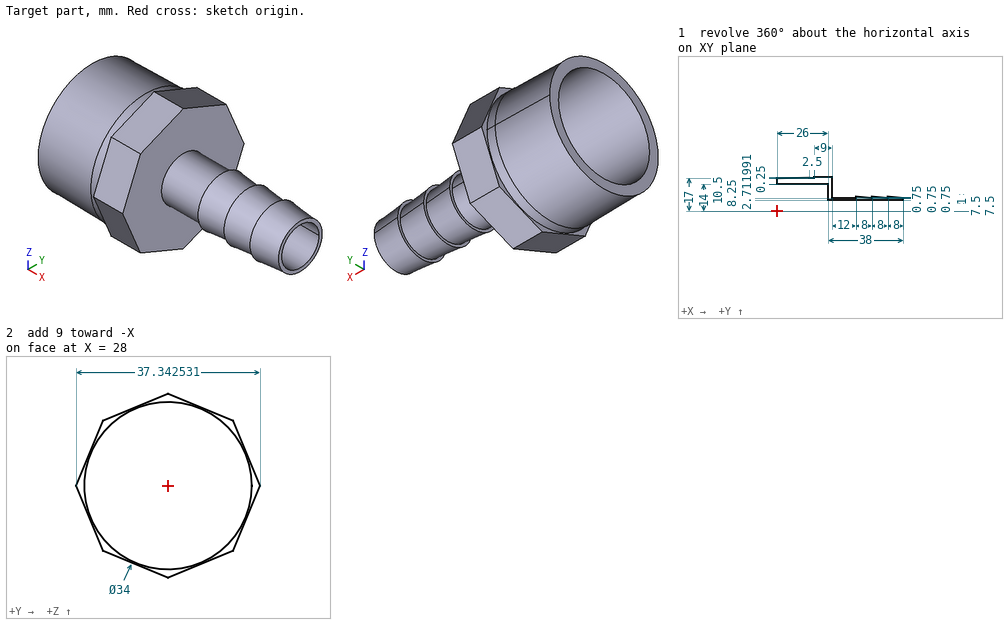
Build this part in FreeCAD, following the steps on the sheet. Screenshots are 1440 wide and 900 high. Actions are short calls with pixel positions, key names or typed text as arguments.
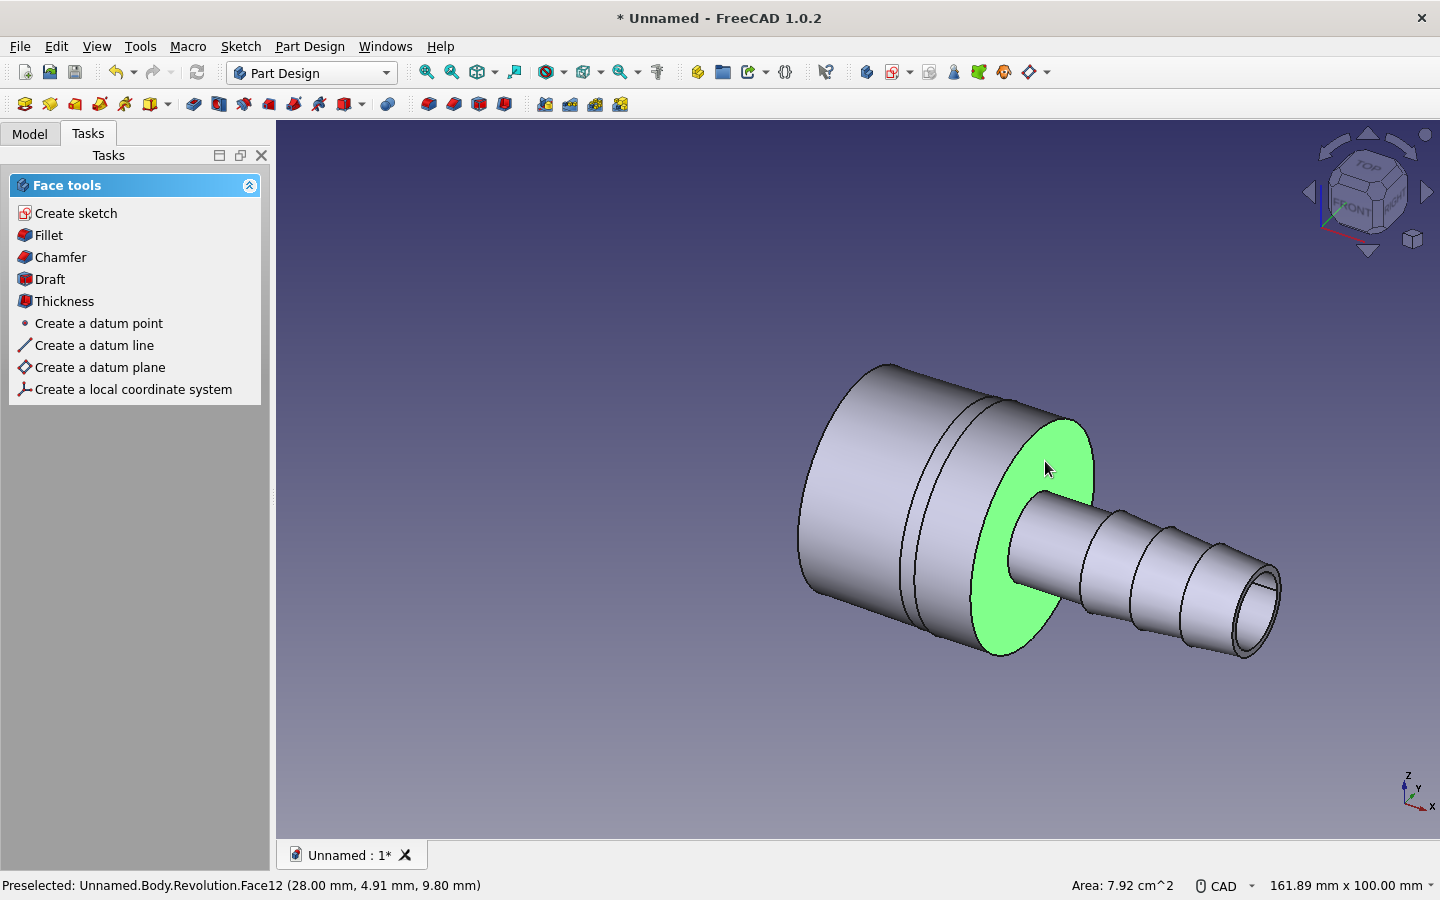
click(892, 72)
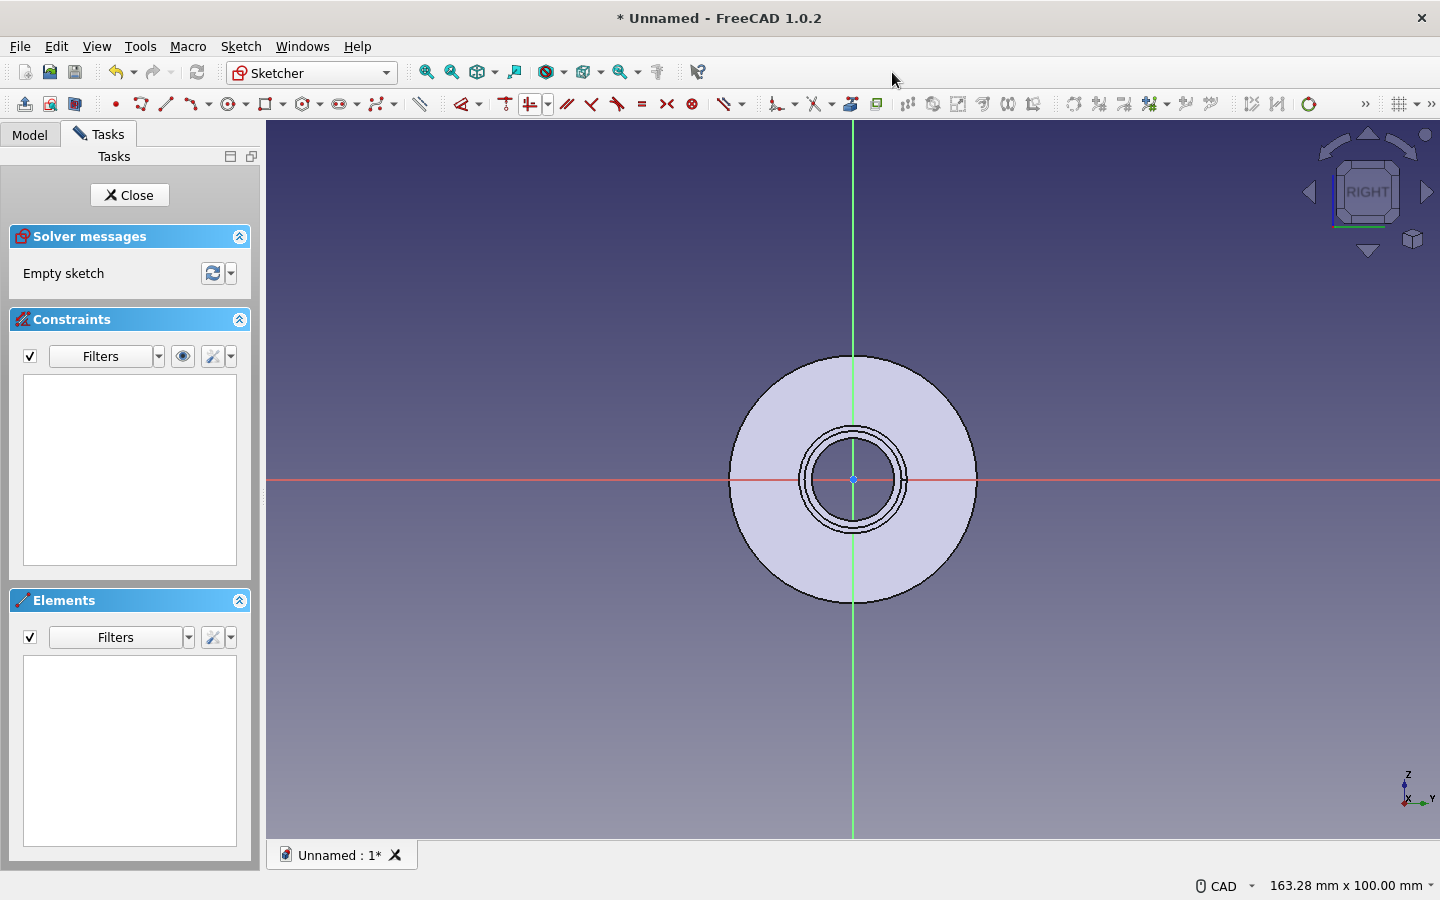
click(75, 104)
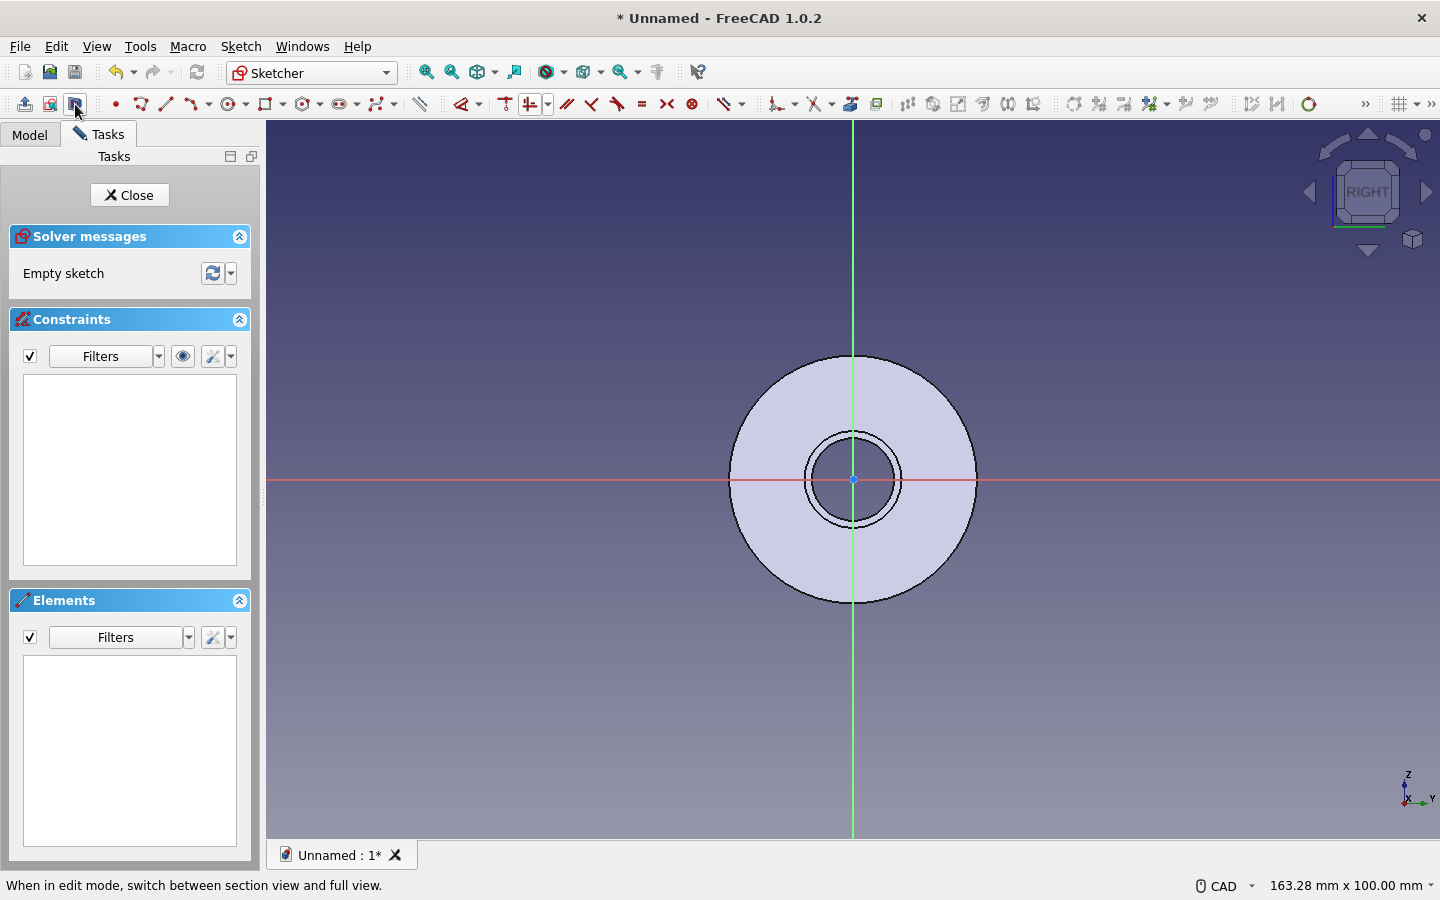
scroll(936, 479, up, 3)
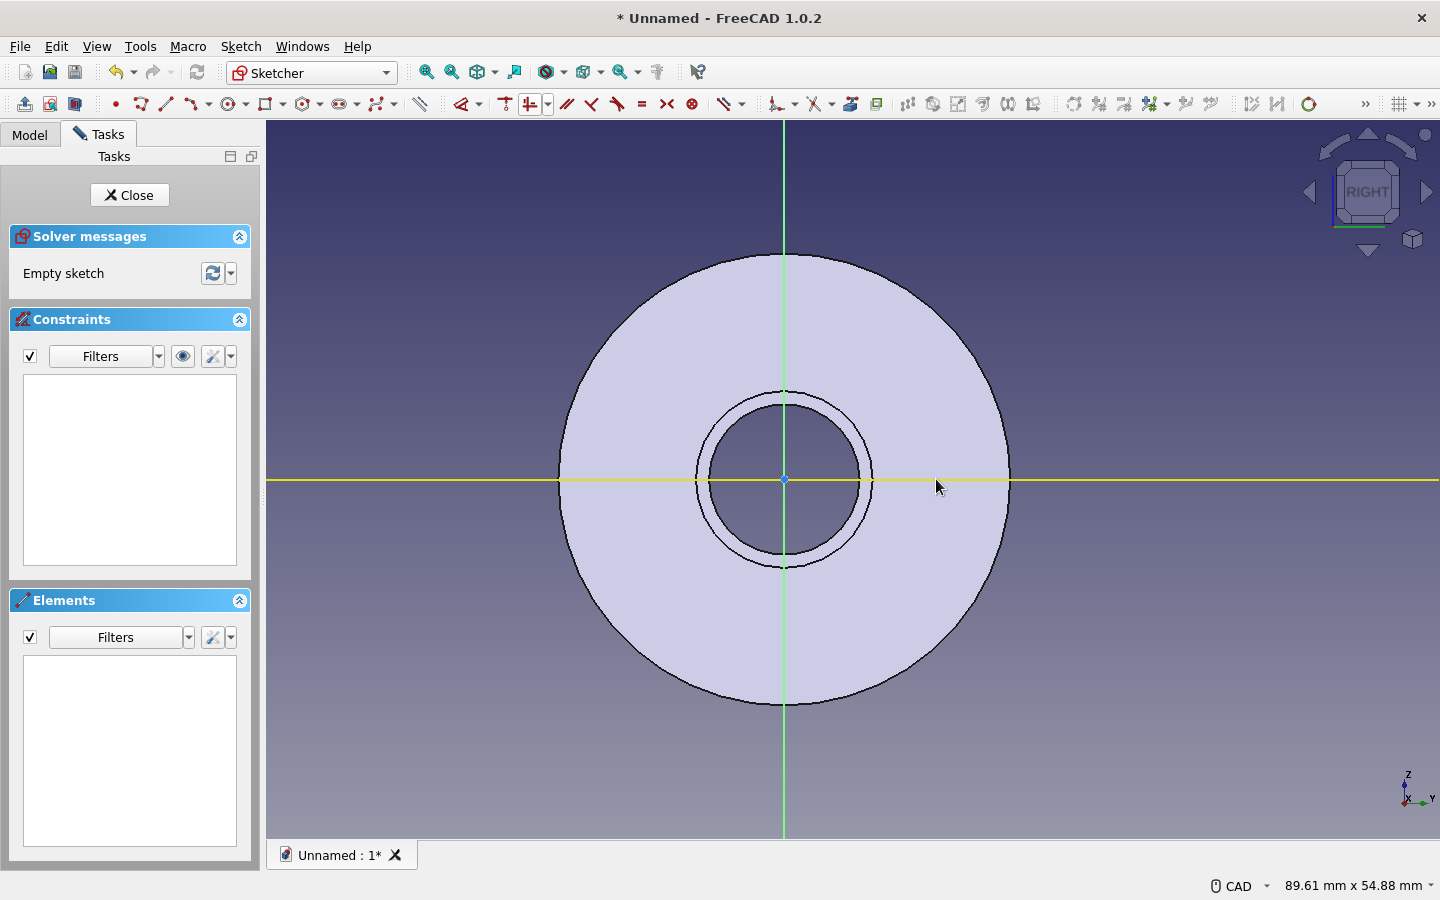
key(g)
key(p)
key(8)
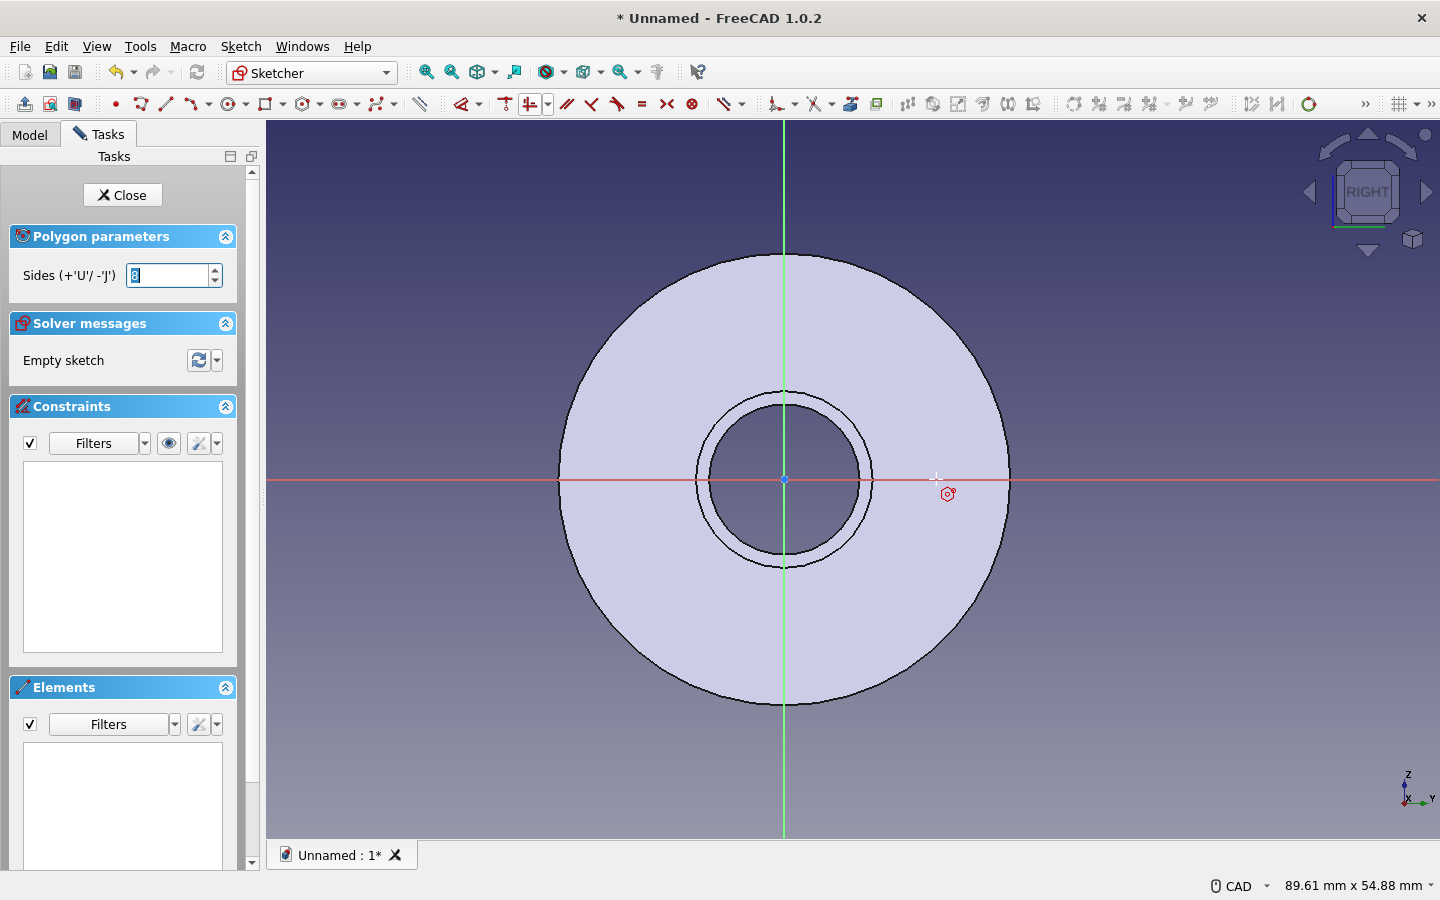
click(784, 479)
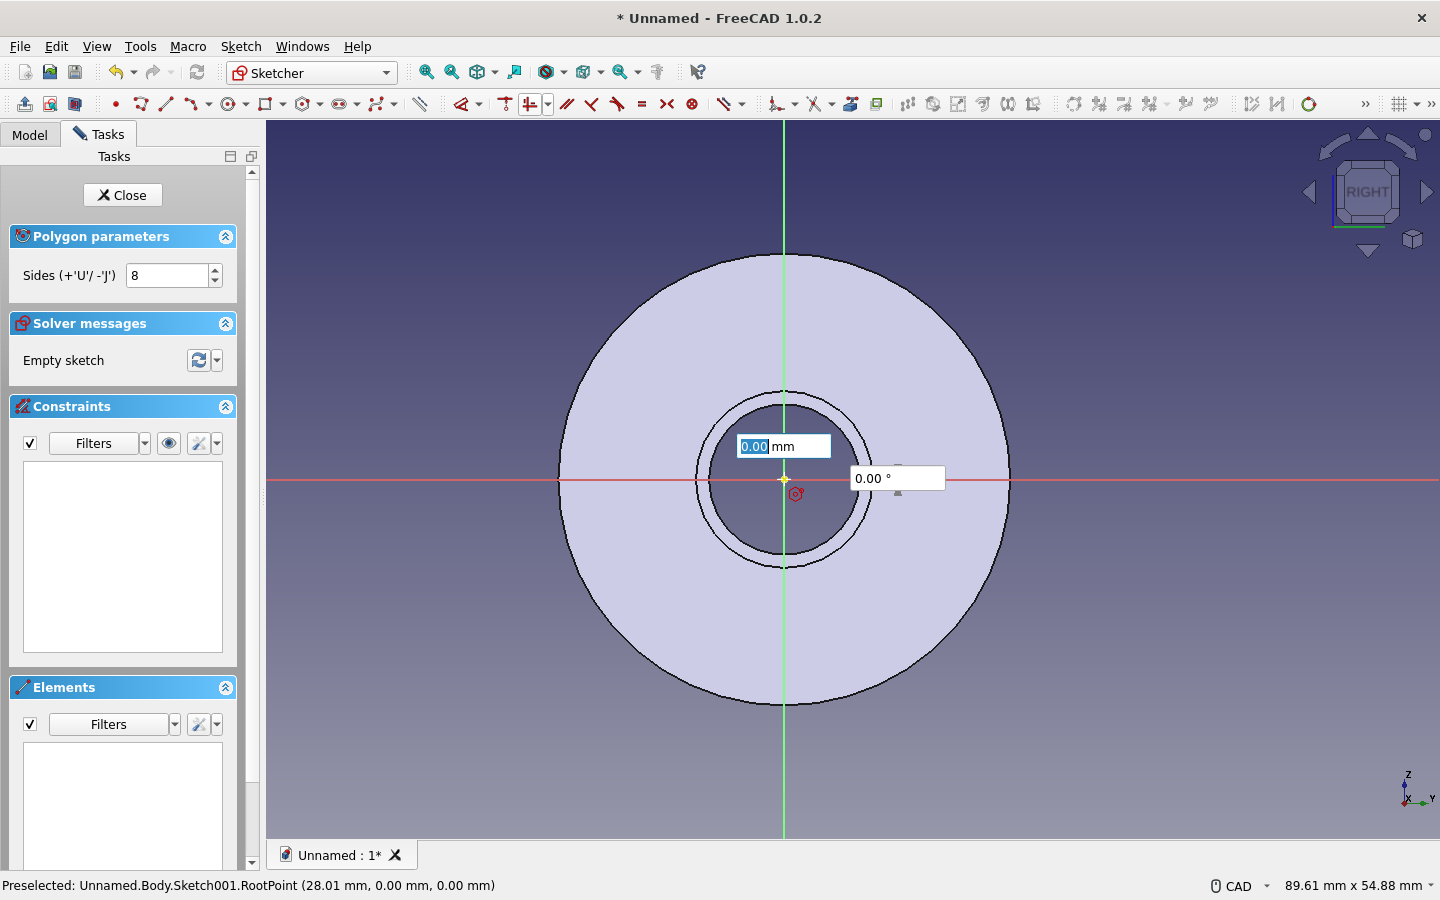
click(1029, 479)
right_click(1029, 479)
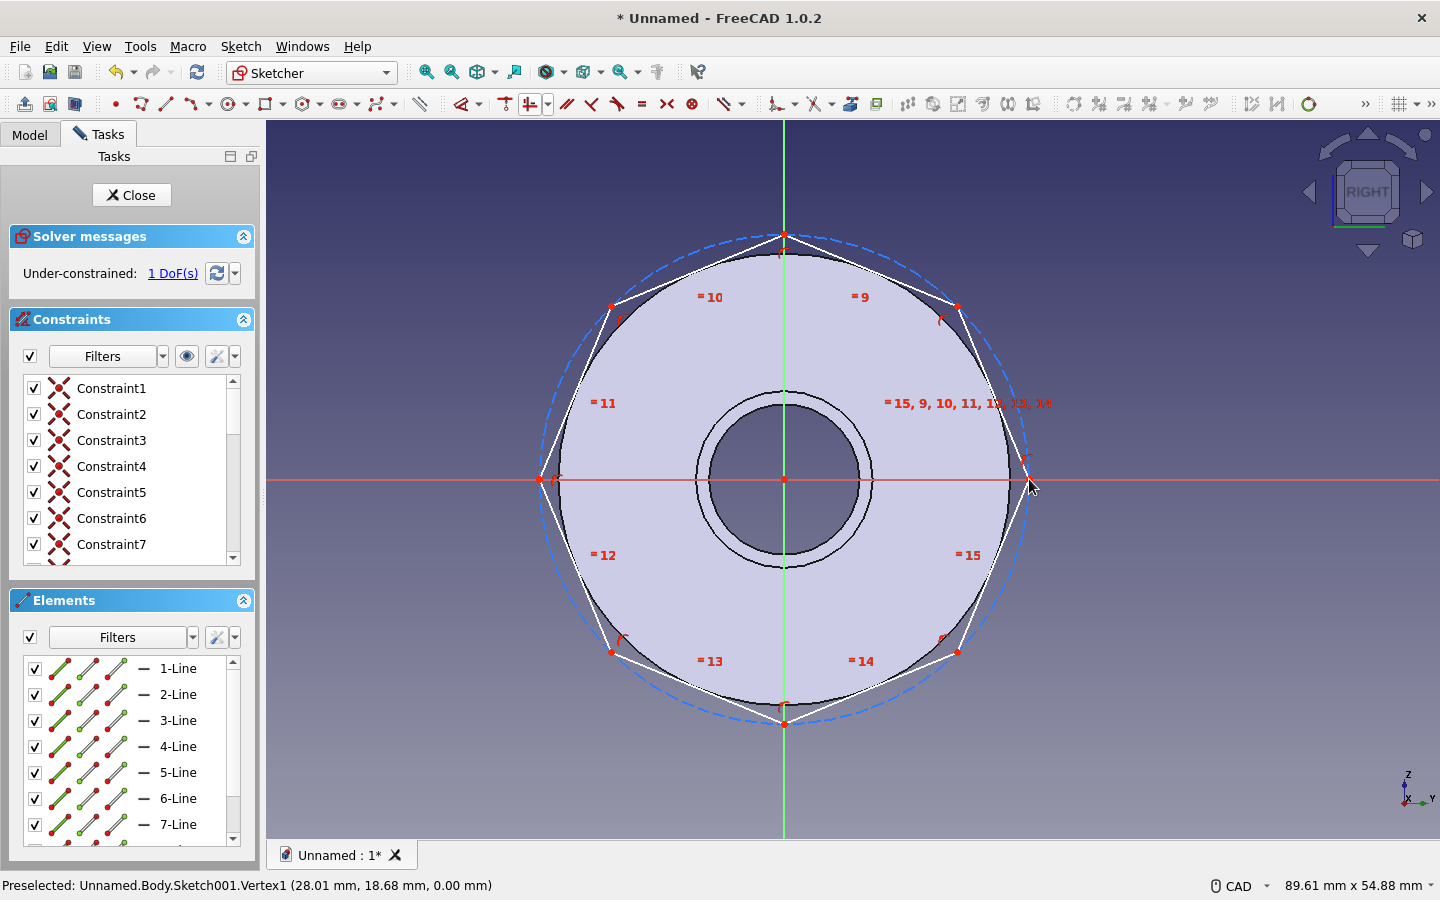
click(228, 104)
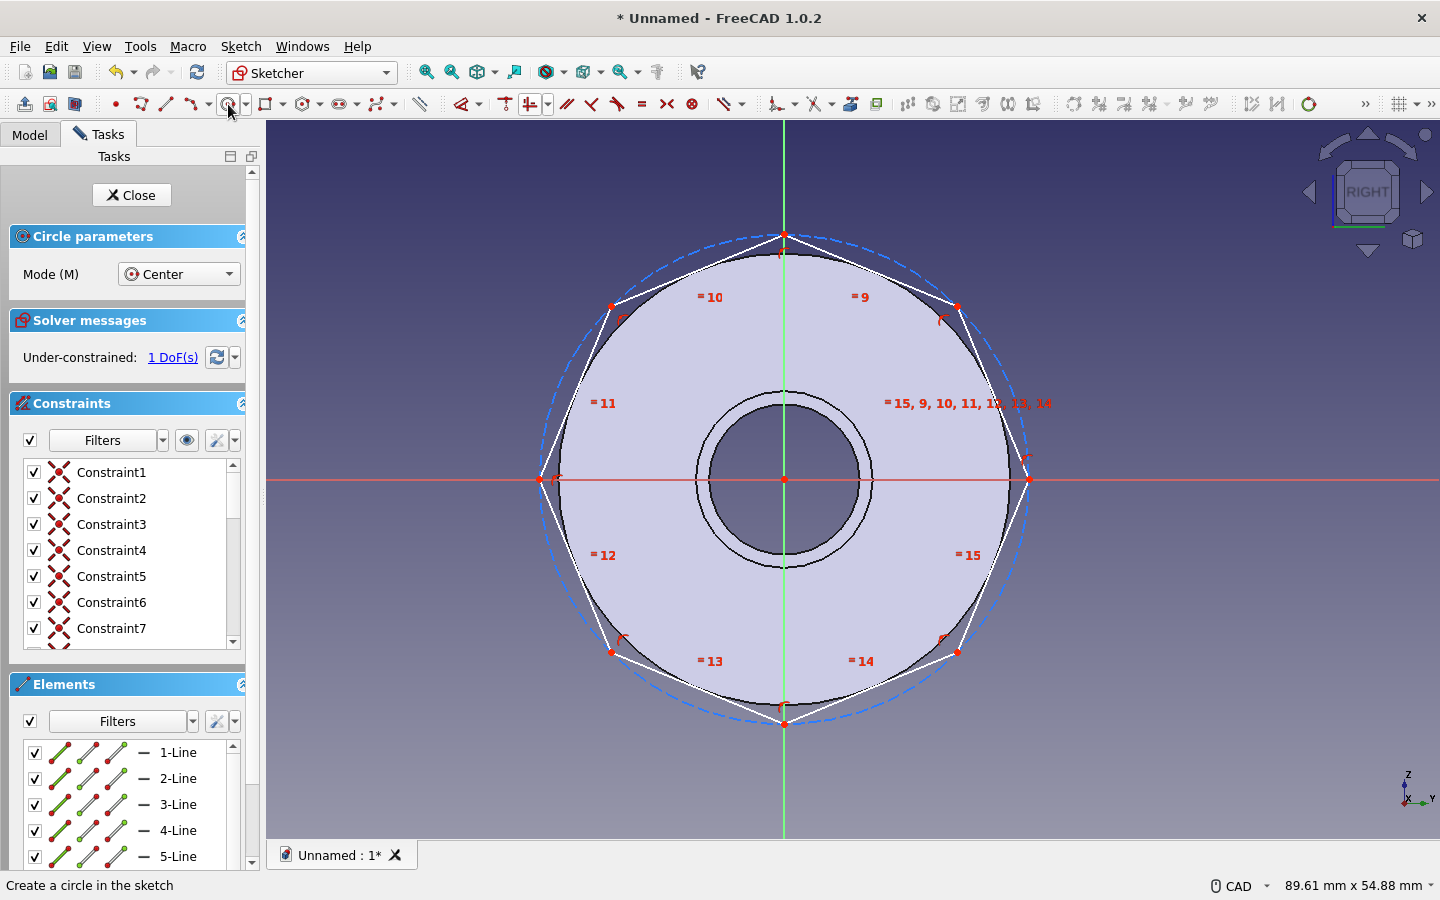
click(784, 479)
click(942, 322)
key(Escape)